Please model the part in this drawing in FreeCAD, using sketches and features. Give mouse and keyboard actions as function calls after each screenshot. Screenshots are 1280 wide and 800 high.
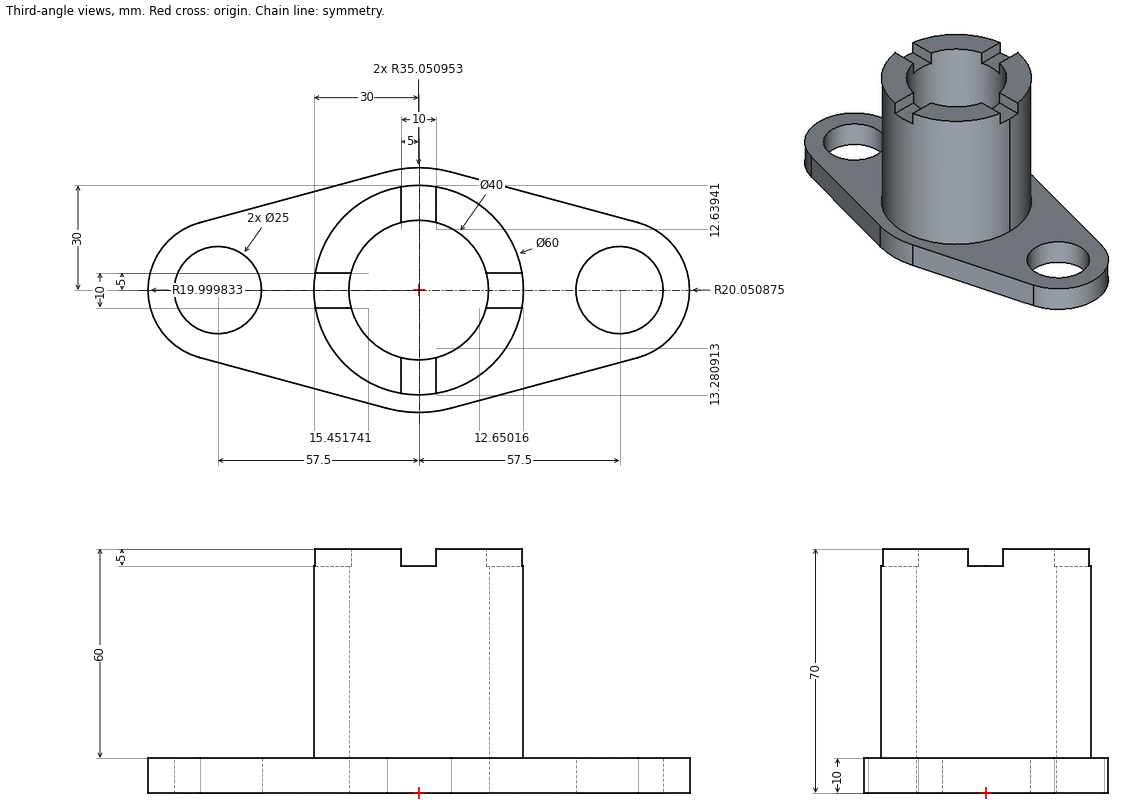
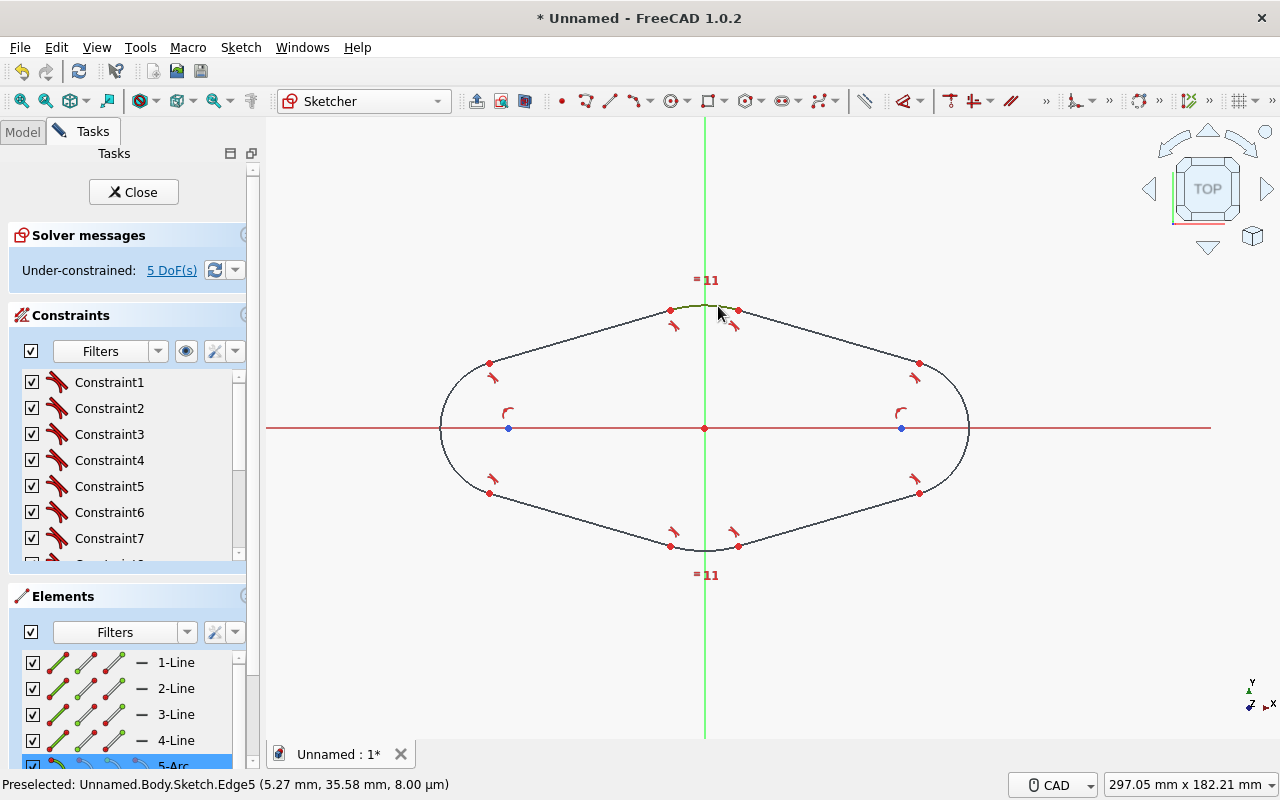
key(k)
key(r)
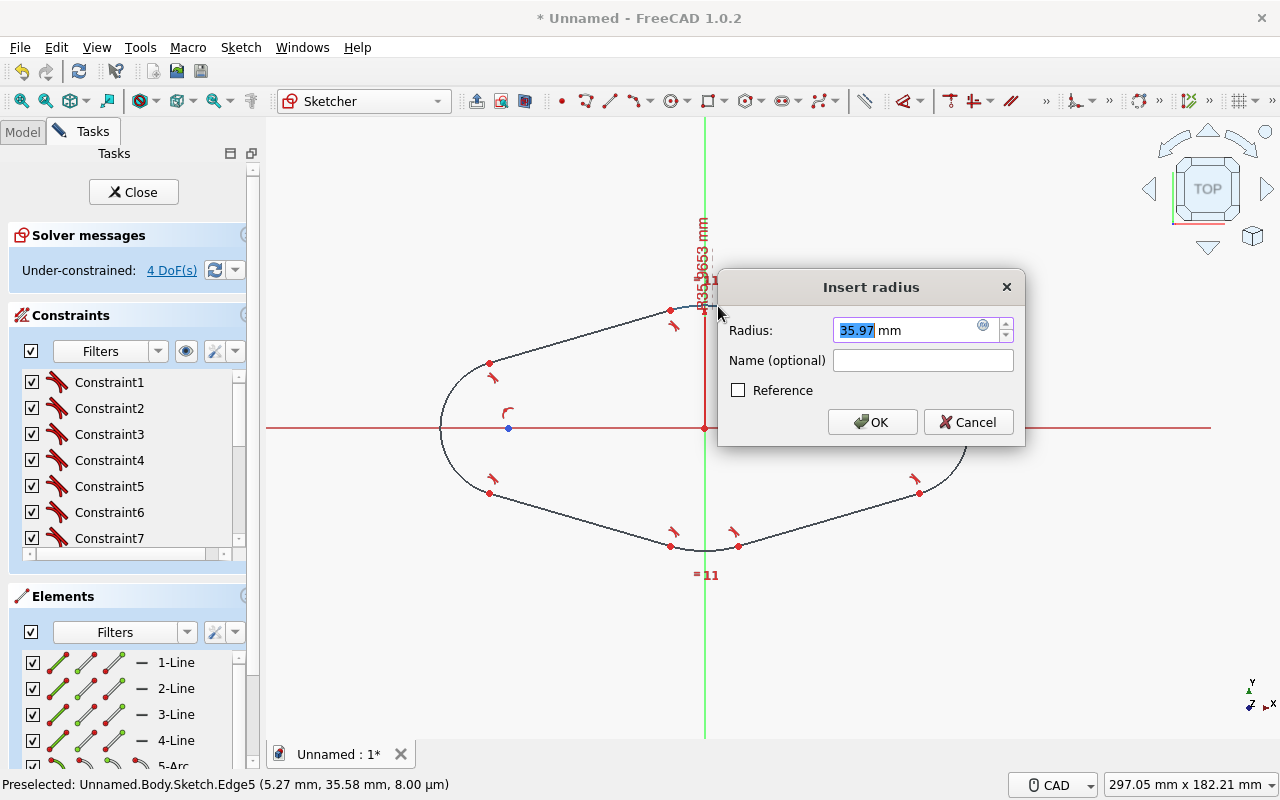
text(35.050953)
key(Return)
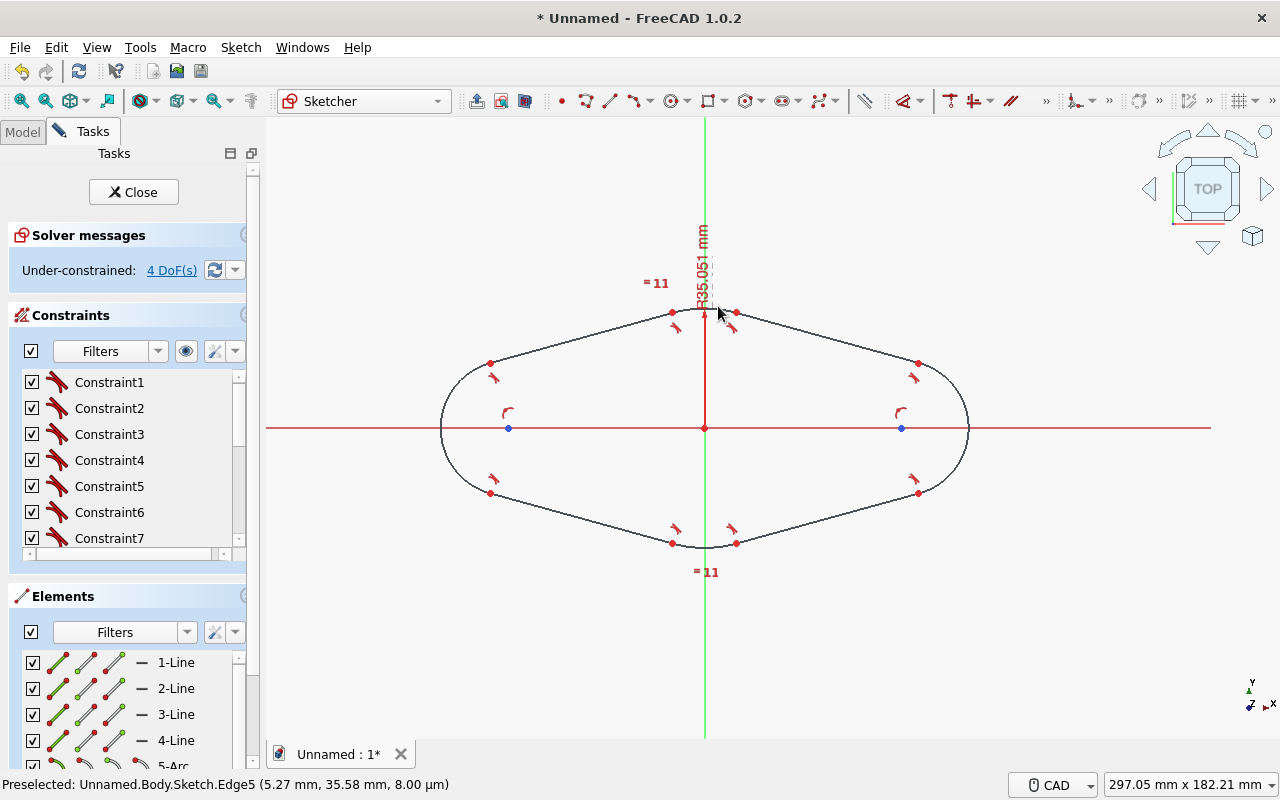
click(450, 395)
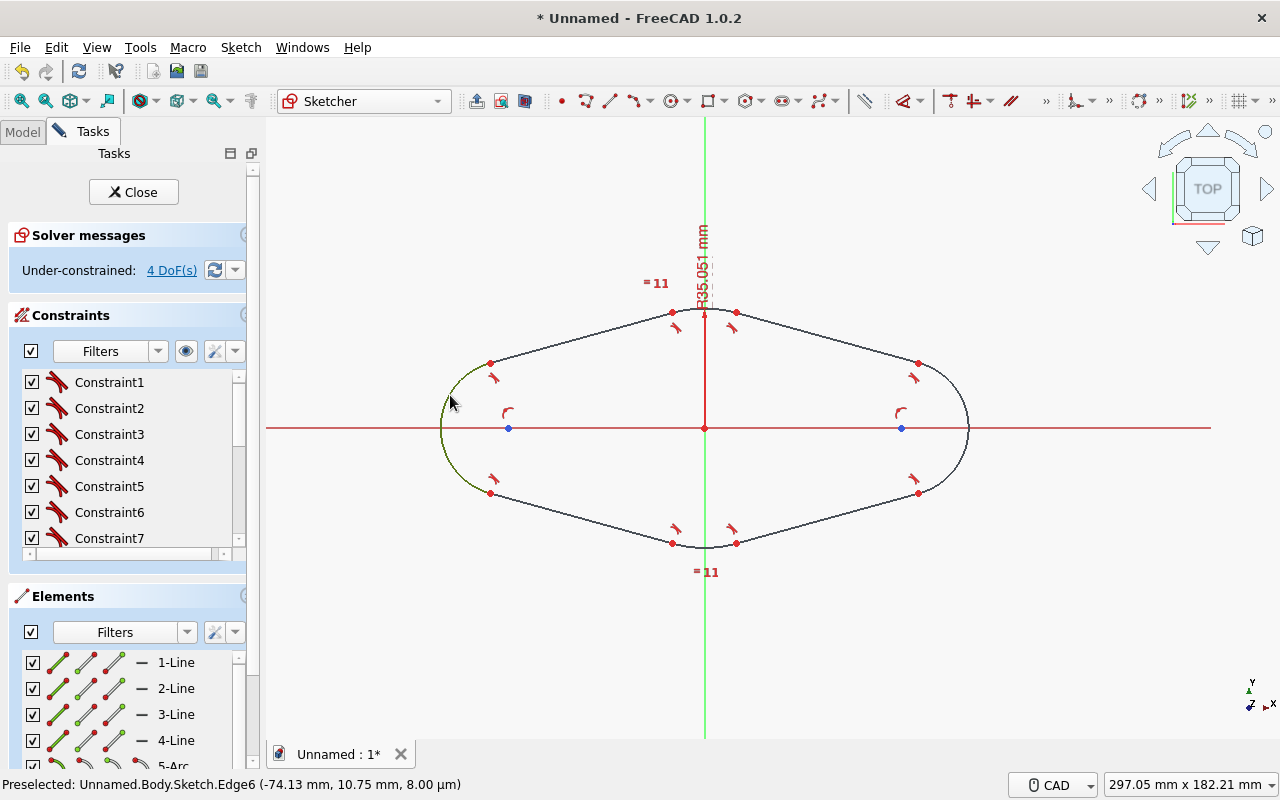
key(k)
key(r)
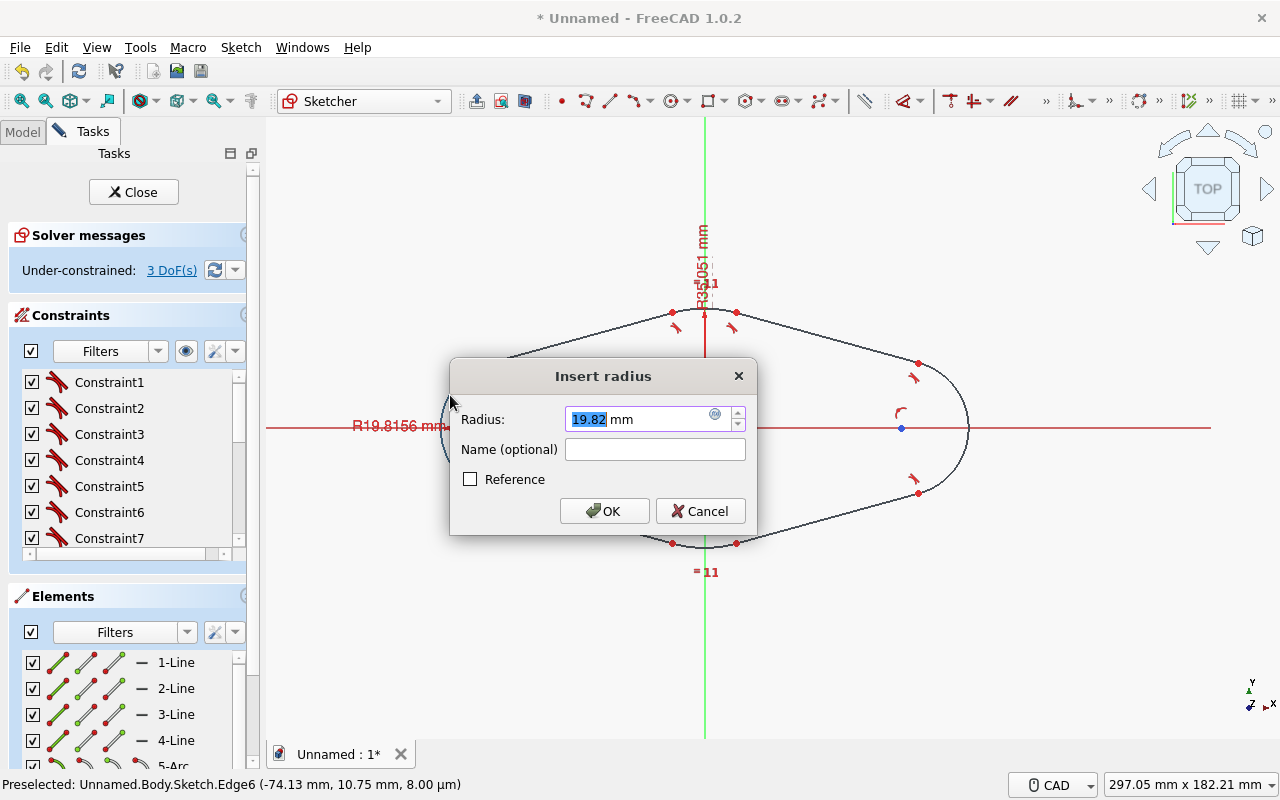
text(19.999833)
key(Return)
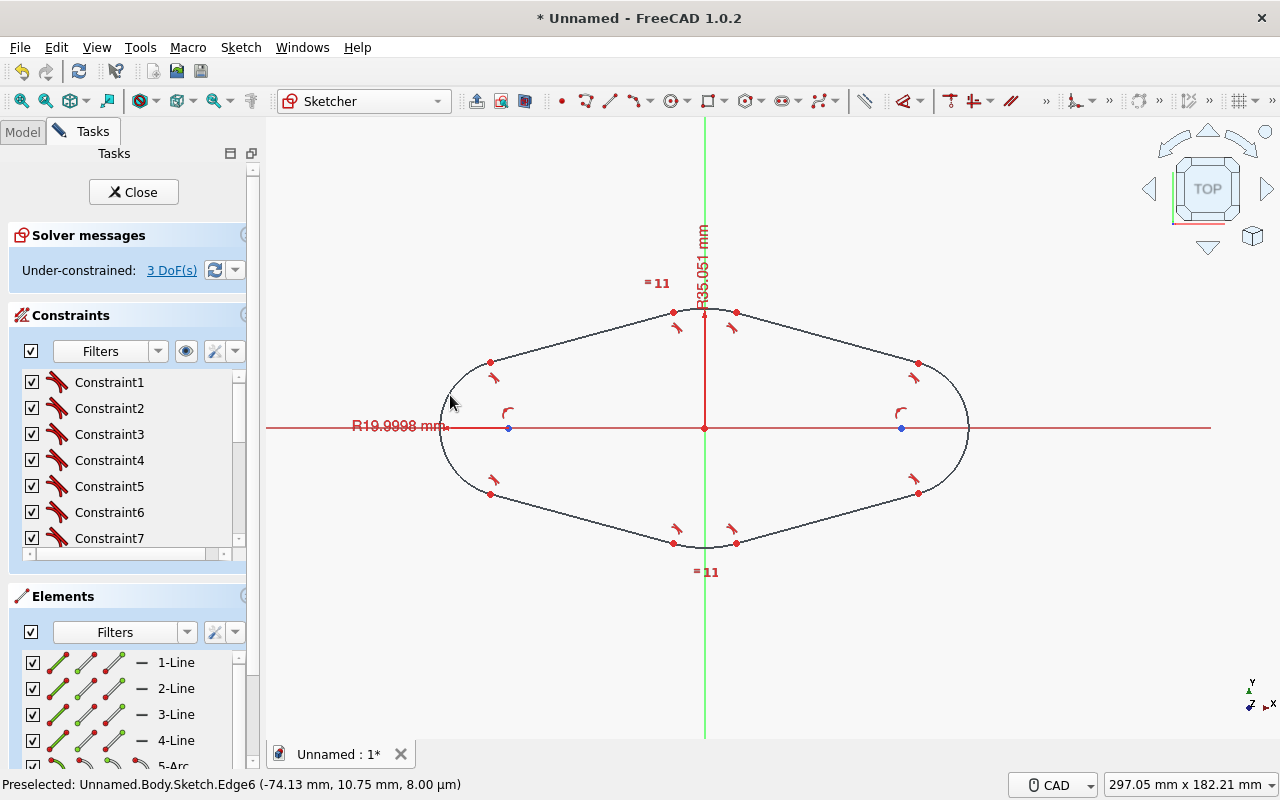
click(960, 462)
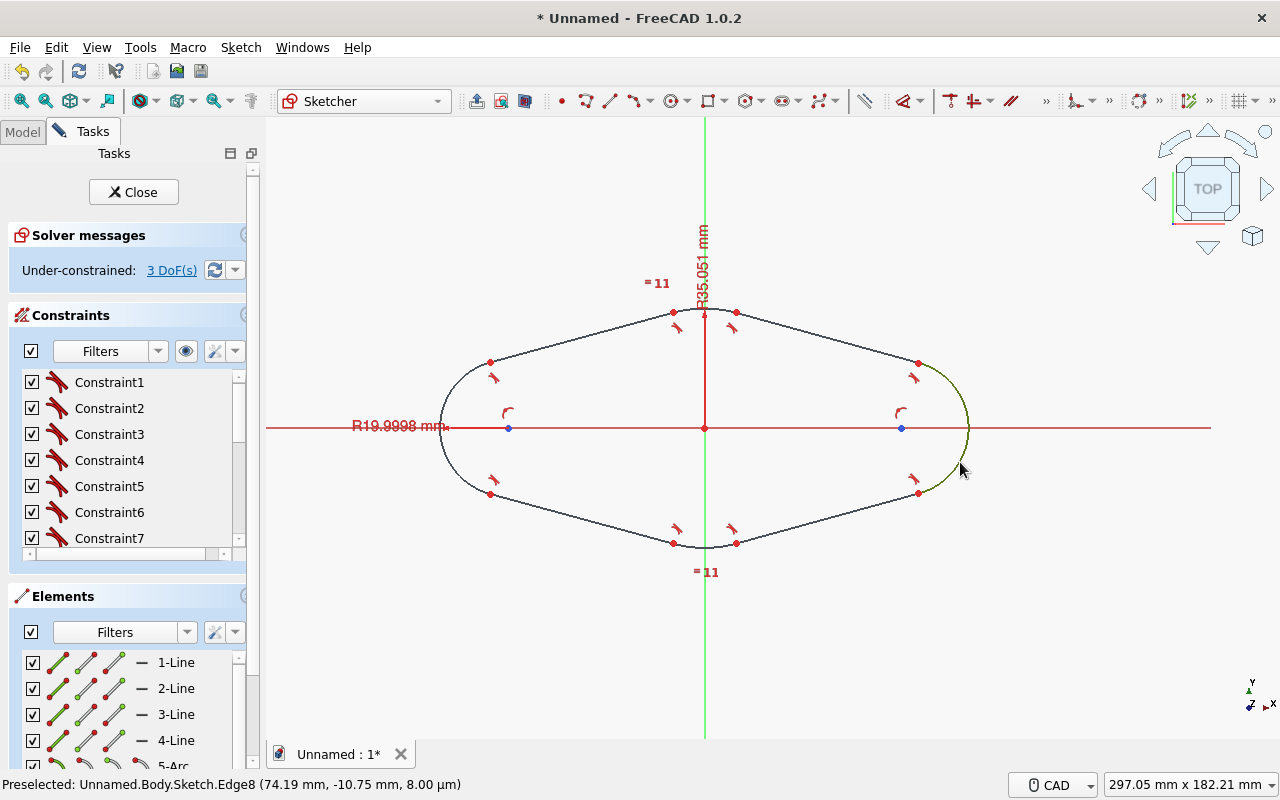
key(k)
key(r)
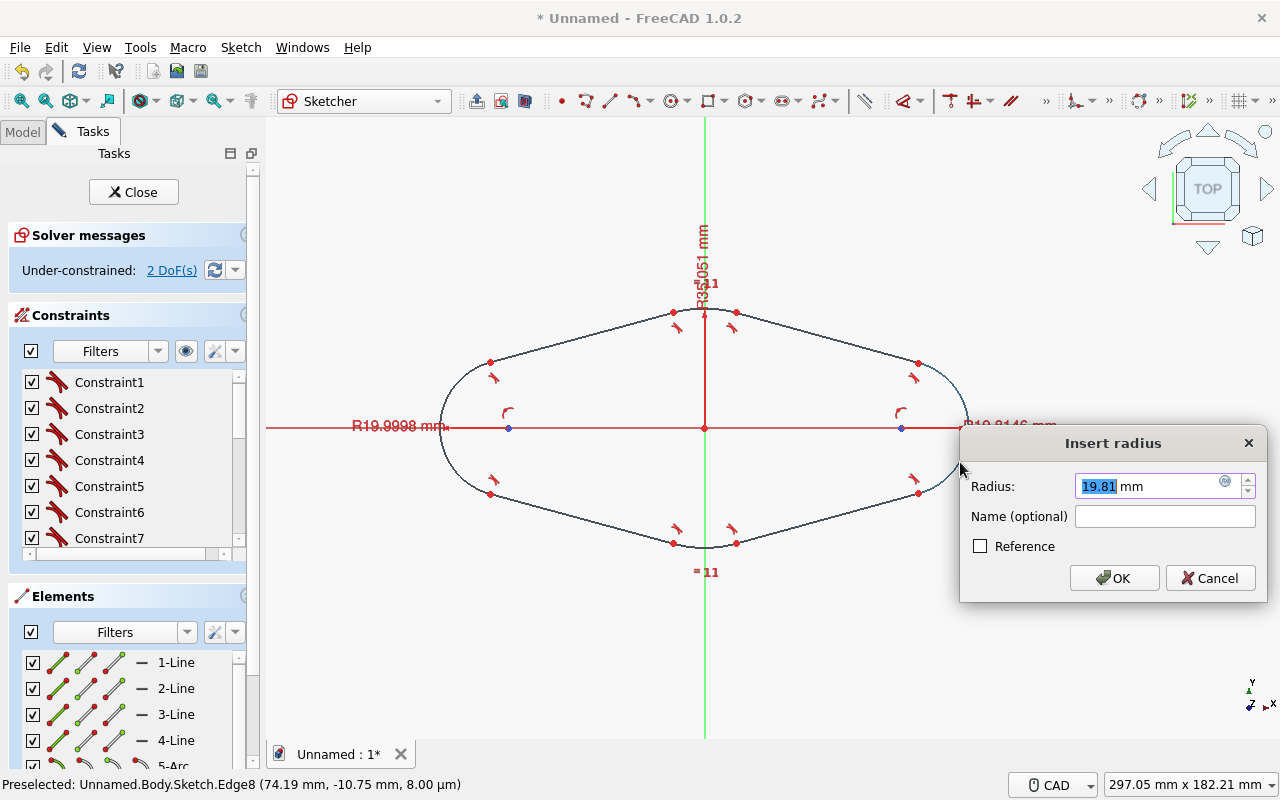
text(20.050875)
key(Return)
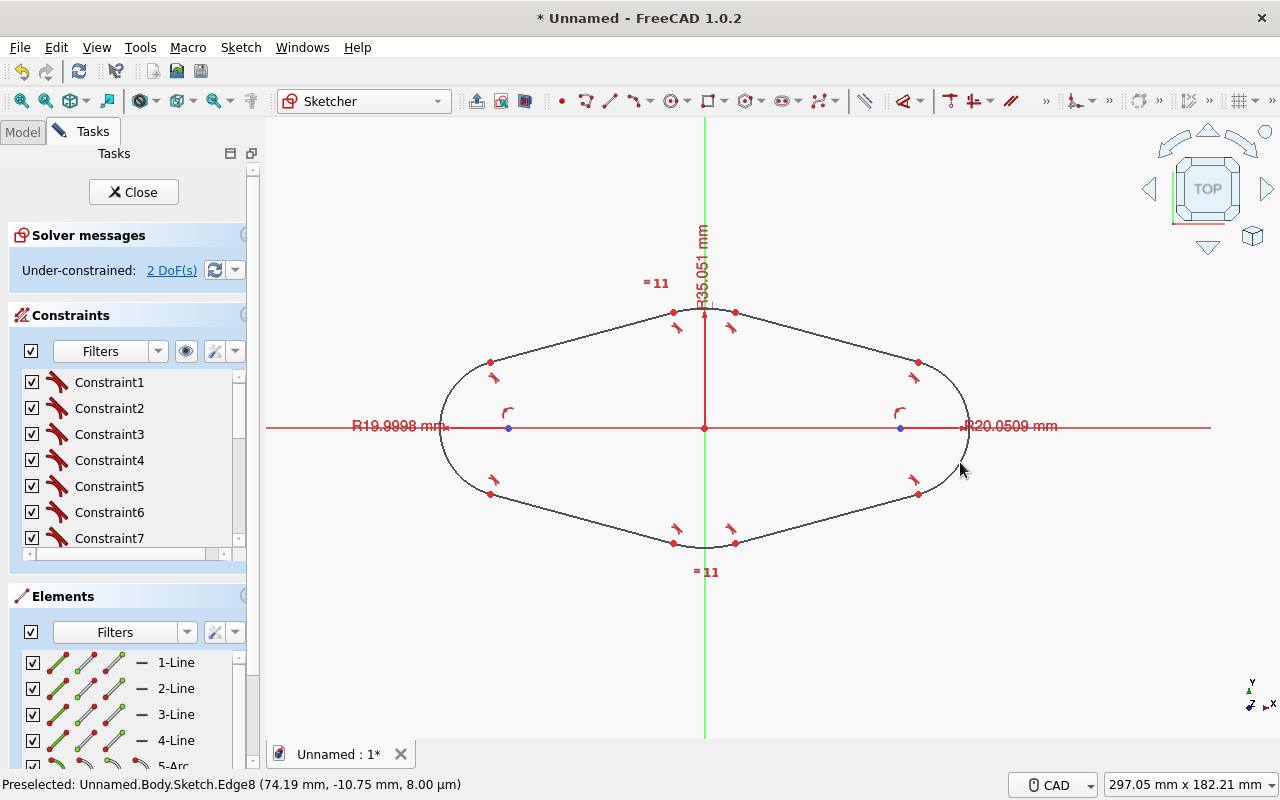
click(508, 428)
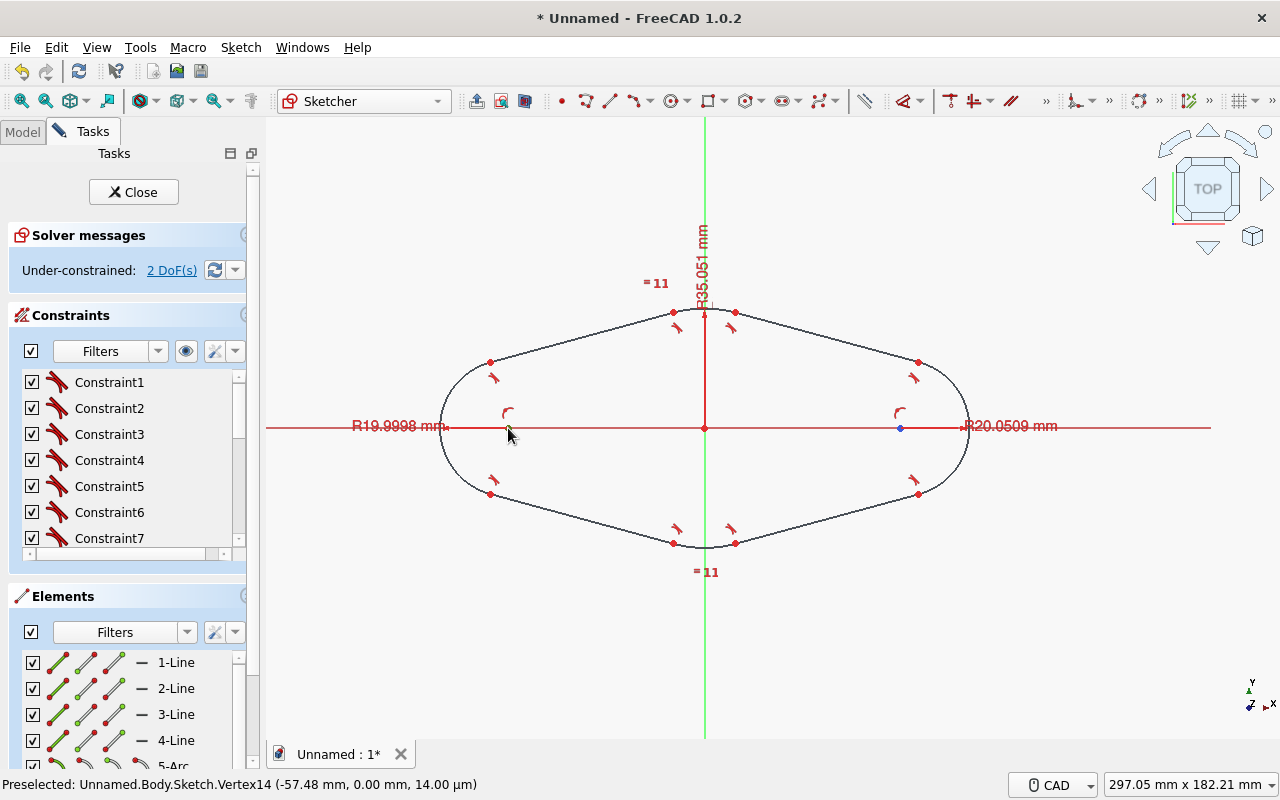
key(l)